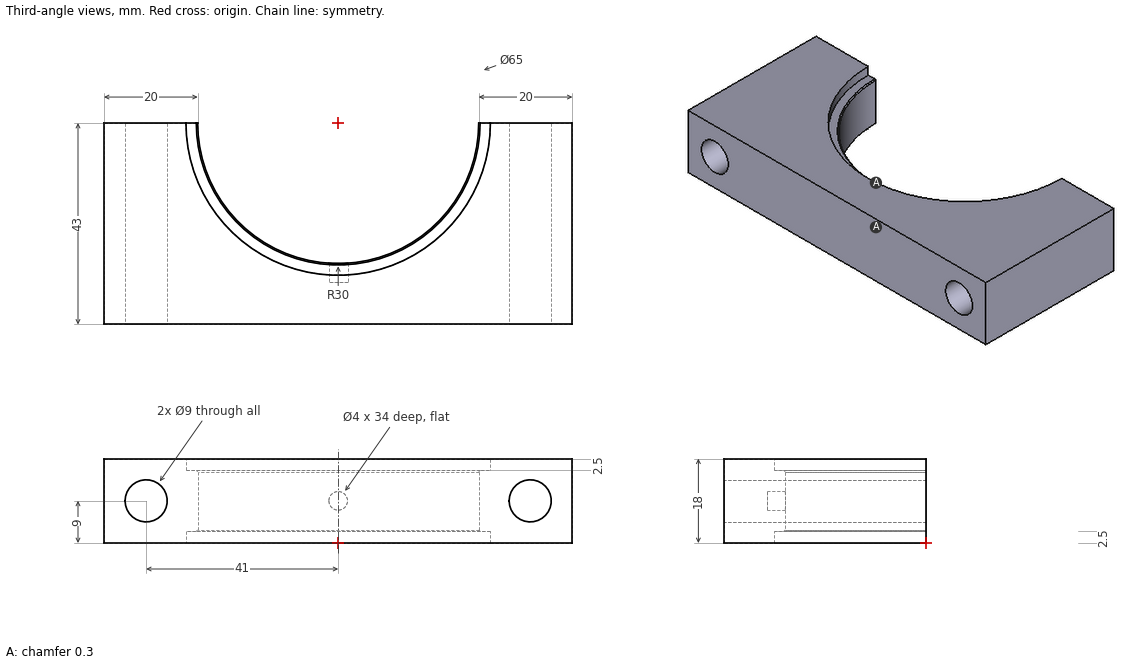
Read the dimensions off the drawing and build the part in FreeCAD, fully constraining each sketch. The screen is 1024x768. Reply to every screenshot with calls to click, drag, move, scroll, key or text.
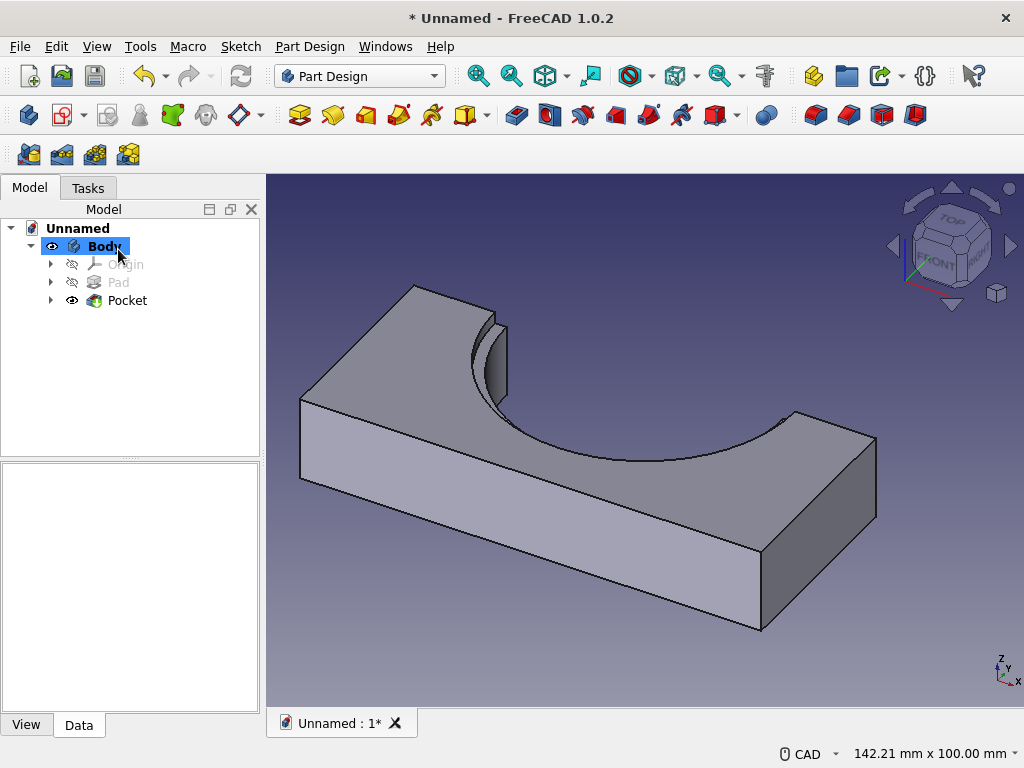
click(51, 264)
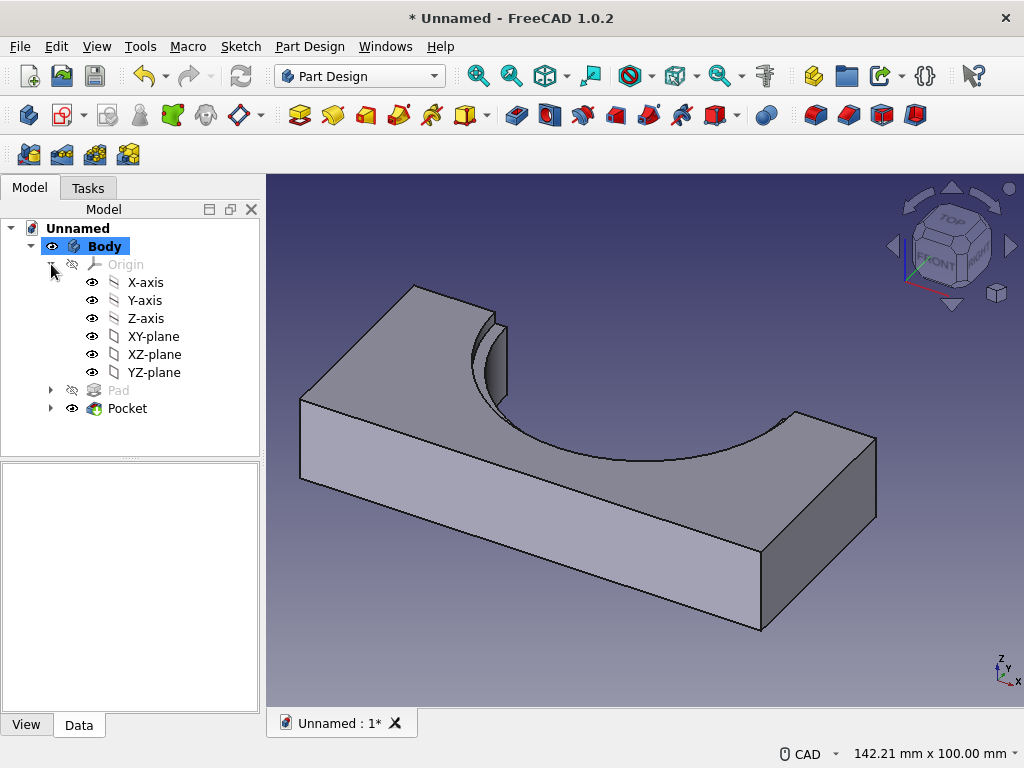
click(137, 336)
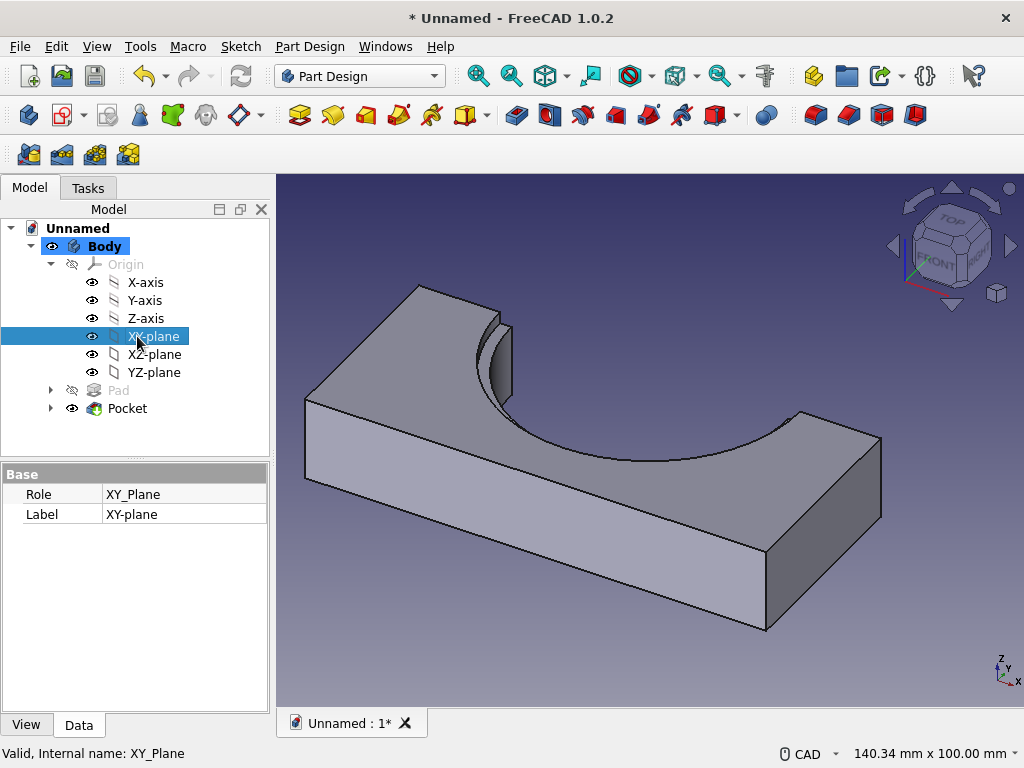
click(238, 116)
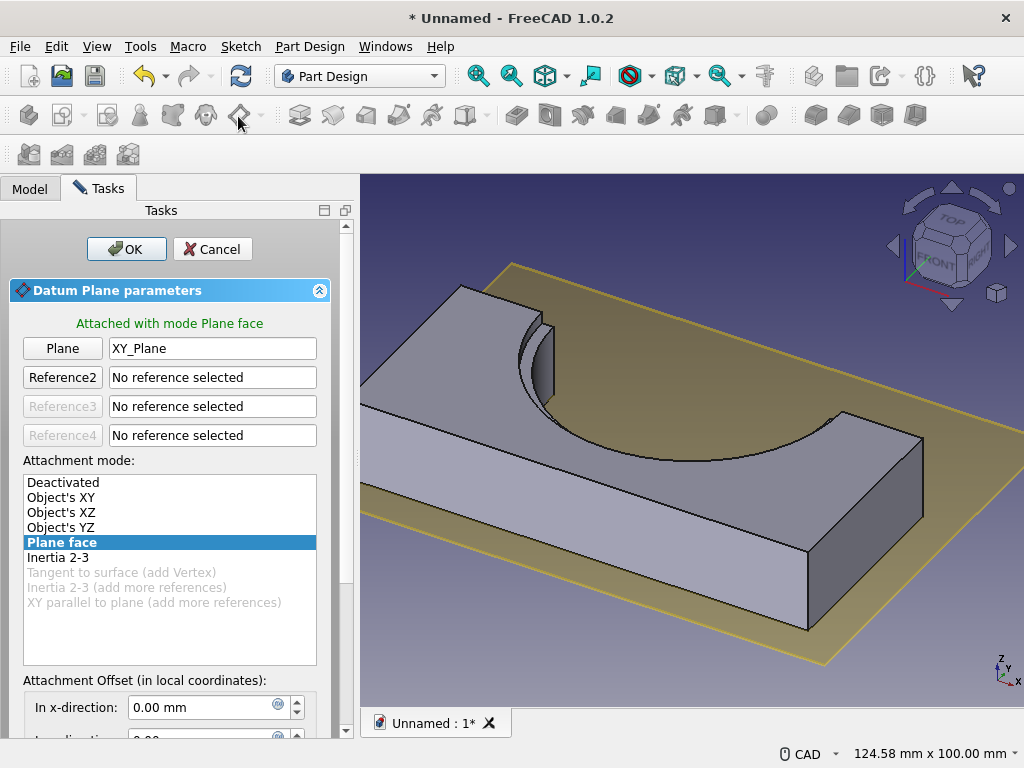
scroll(346, 479, down, 2)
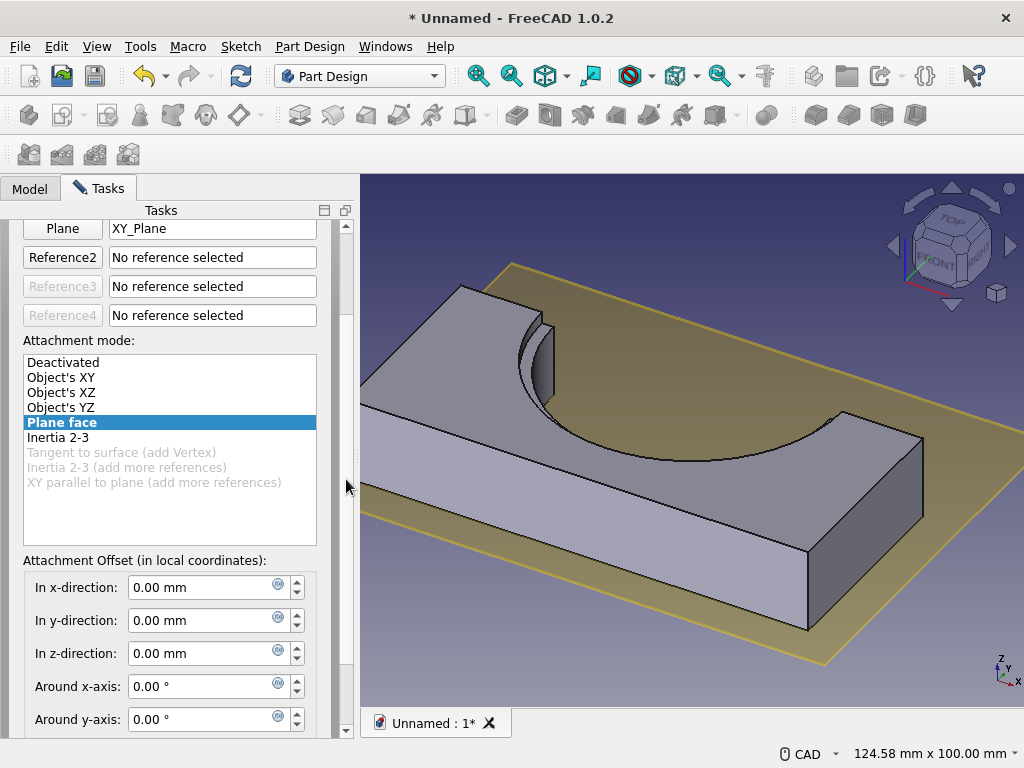
triple_click(210, 654)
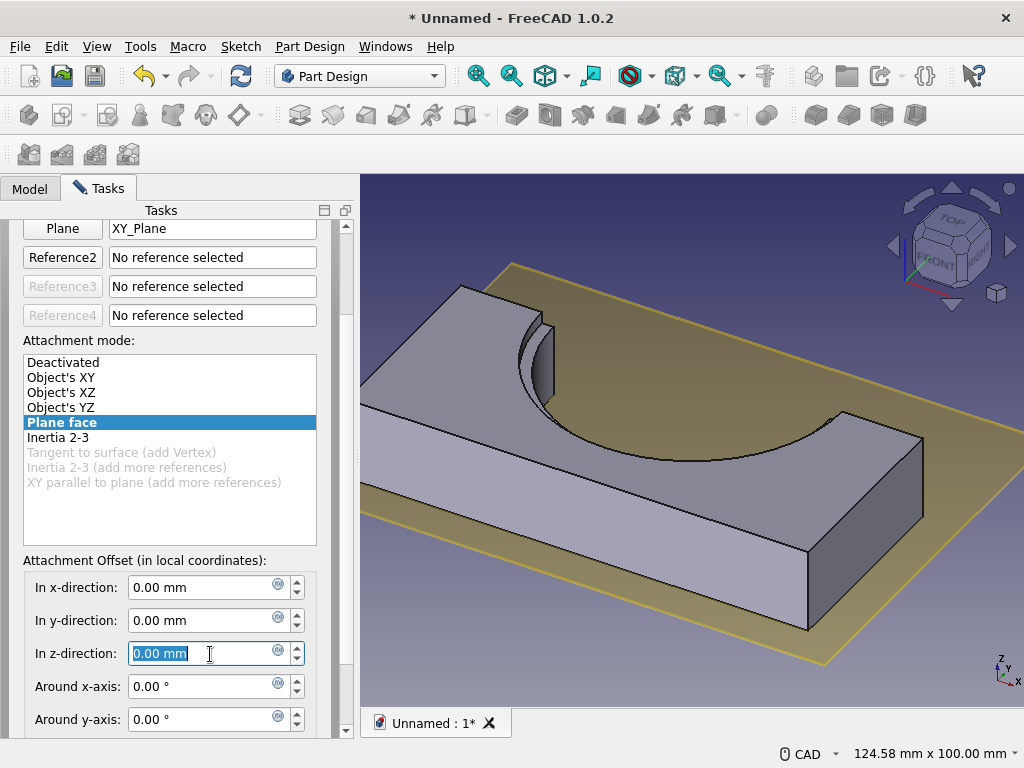
text(2.5)
key(Tab)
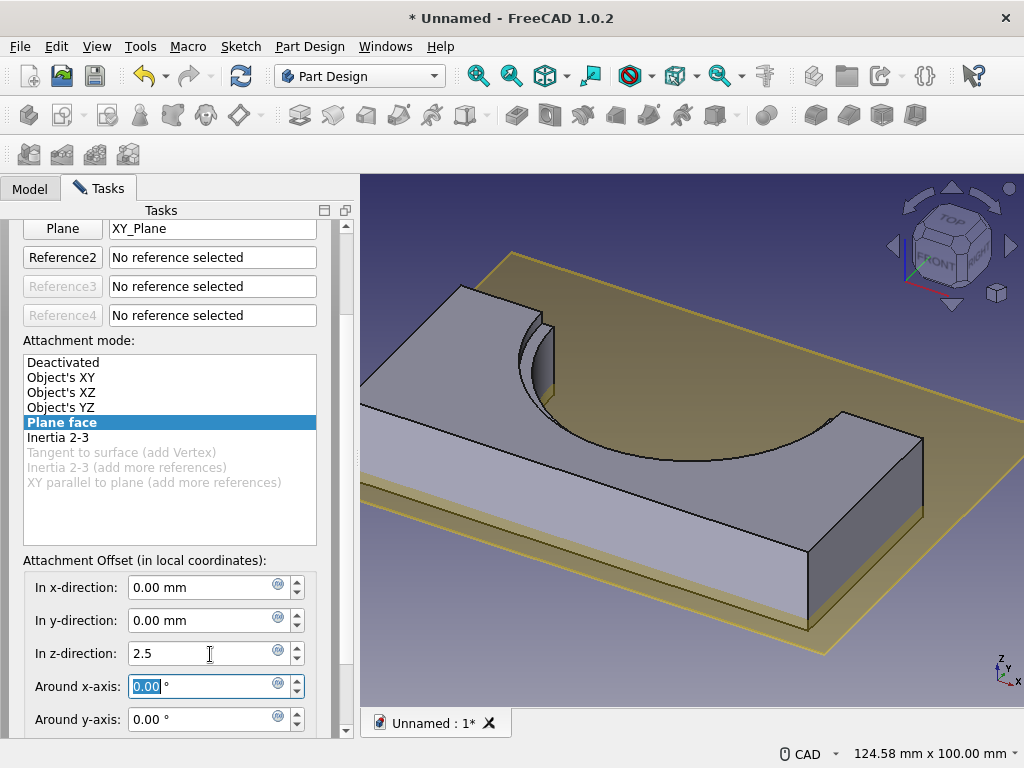
scroll(346, 479, up, 3)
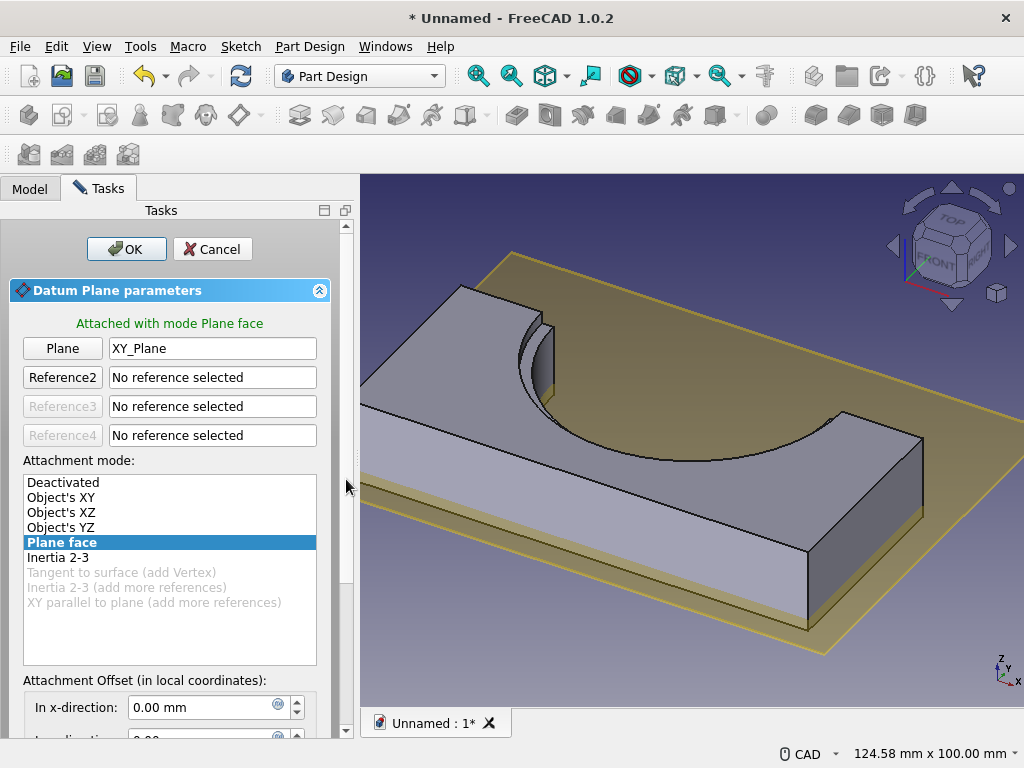
click(127, 249)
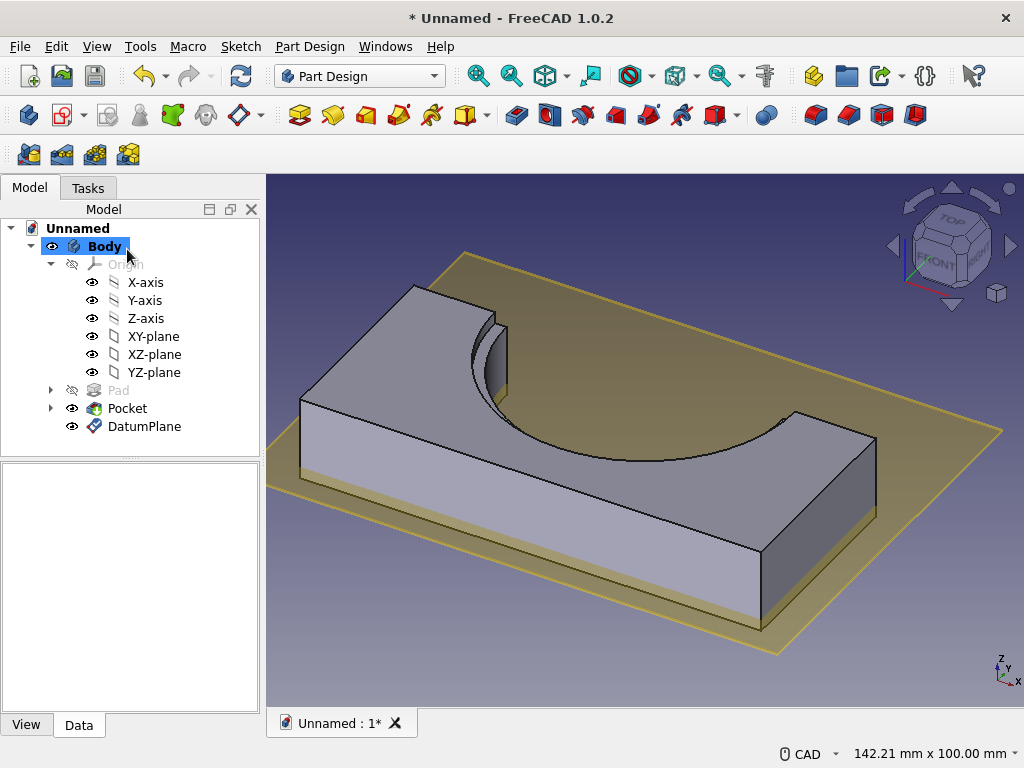
click(117, 426)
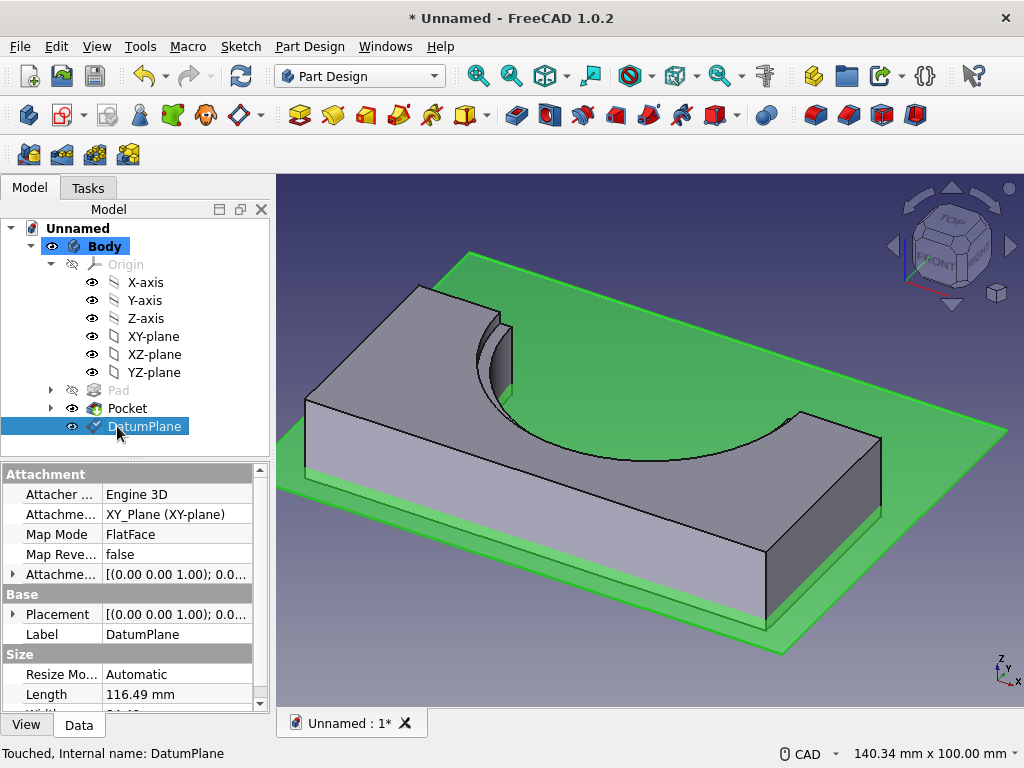
click(62, 116)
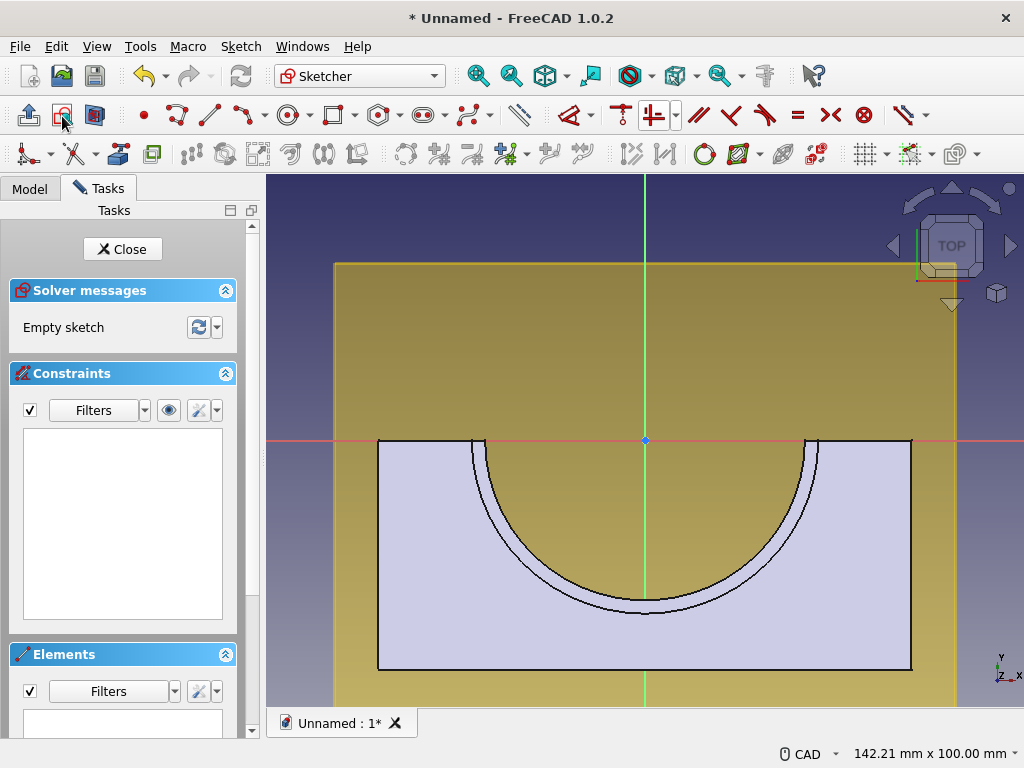
click(95, 116)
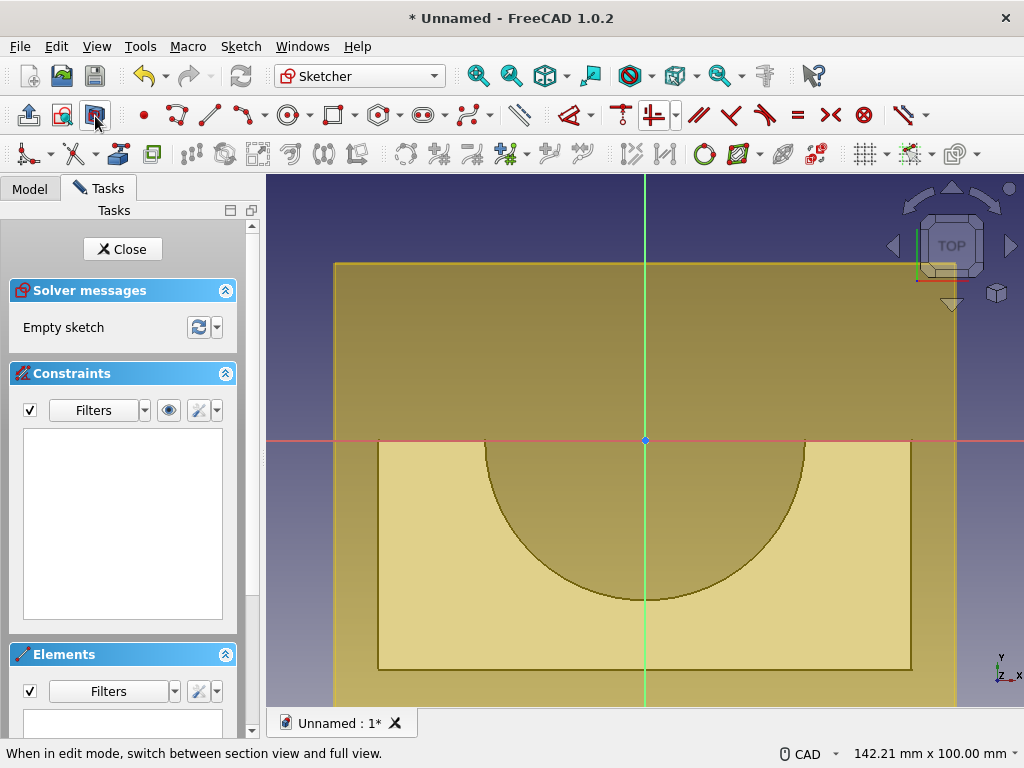
click(288, 116)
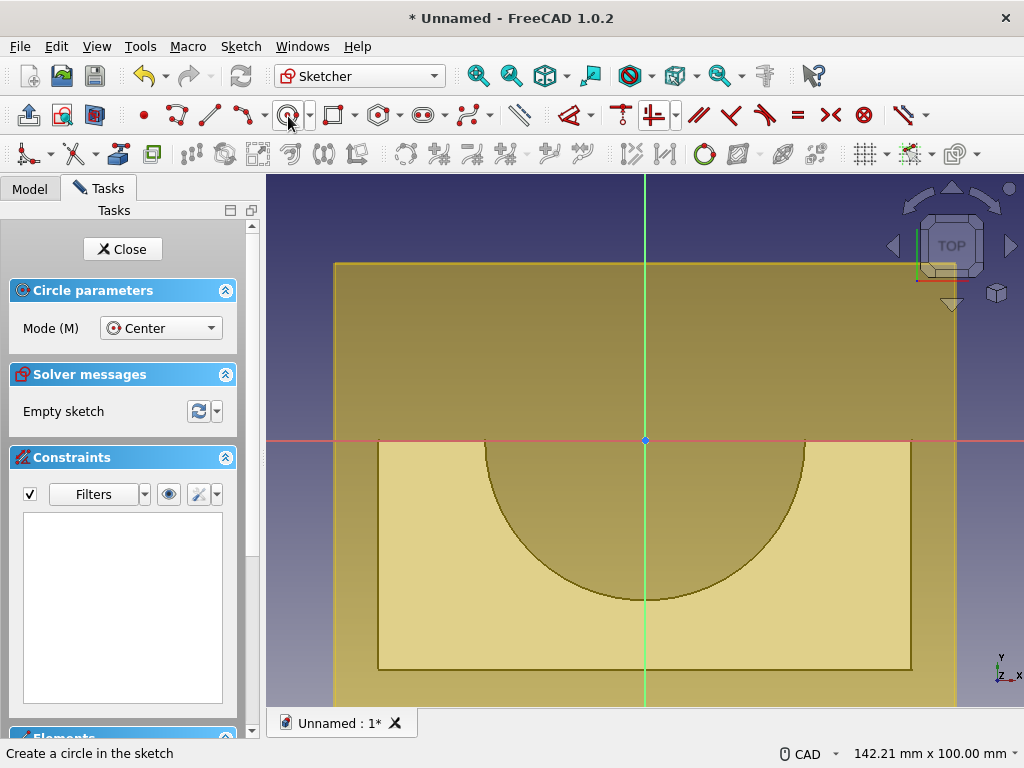
click(645, 440)
move(767, 318)